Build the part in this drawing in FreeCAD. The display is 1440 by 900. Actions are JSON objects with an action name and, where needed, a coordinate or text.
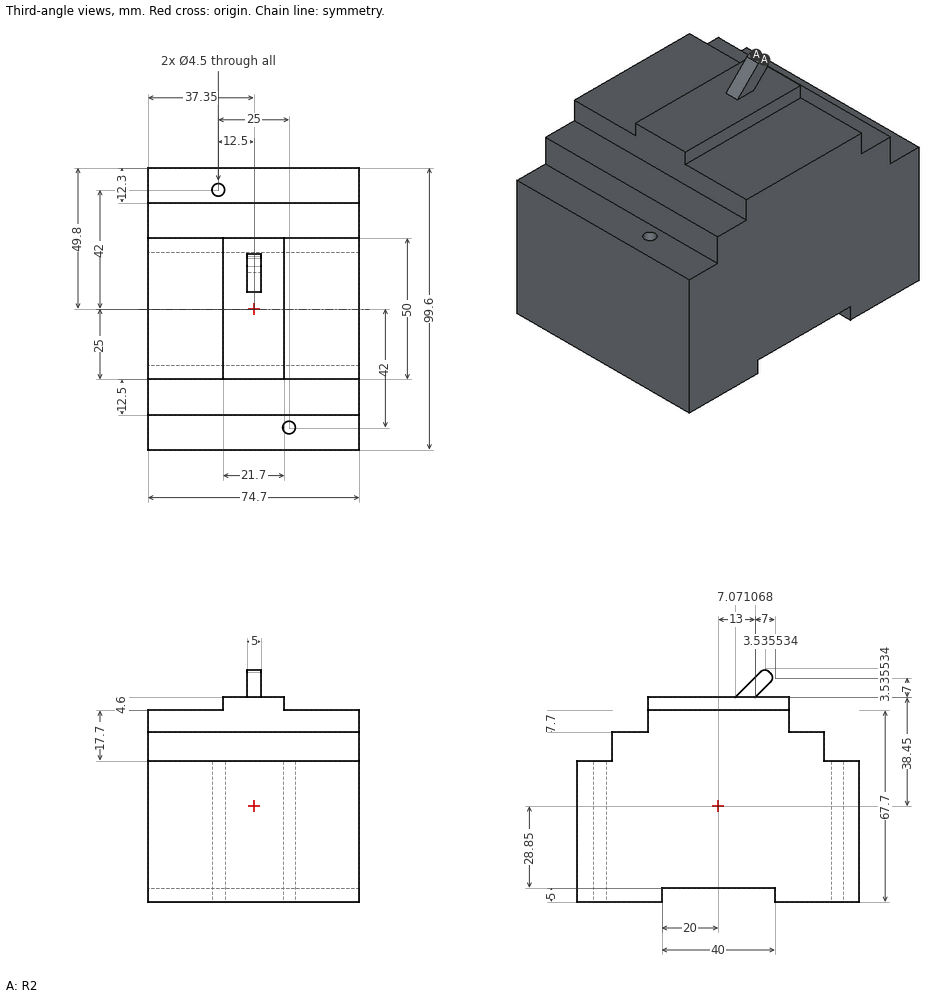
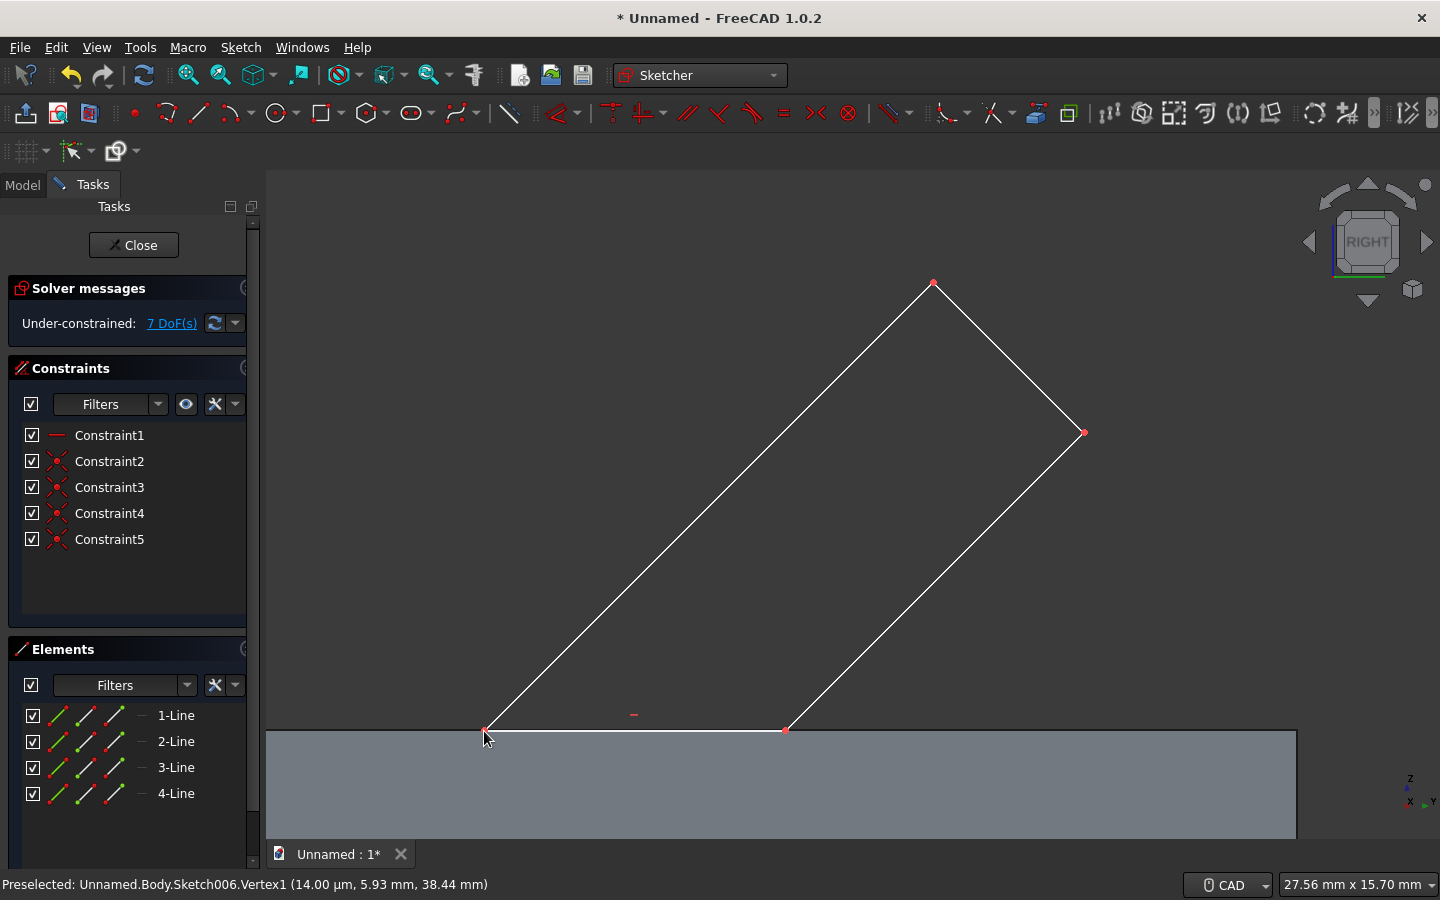
{"action": "left_click", "coordinate": [556, 114]}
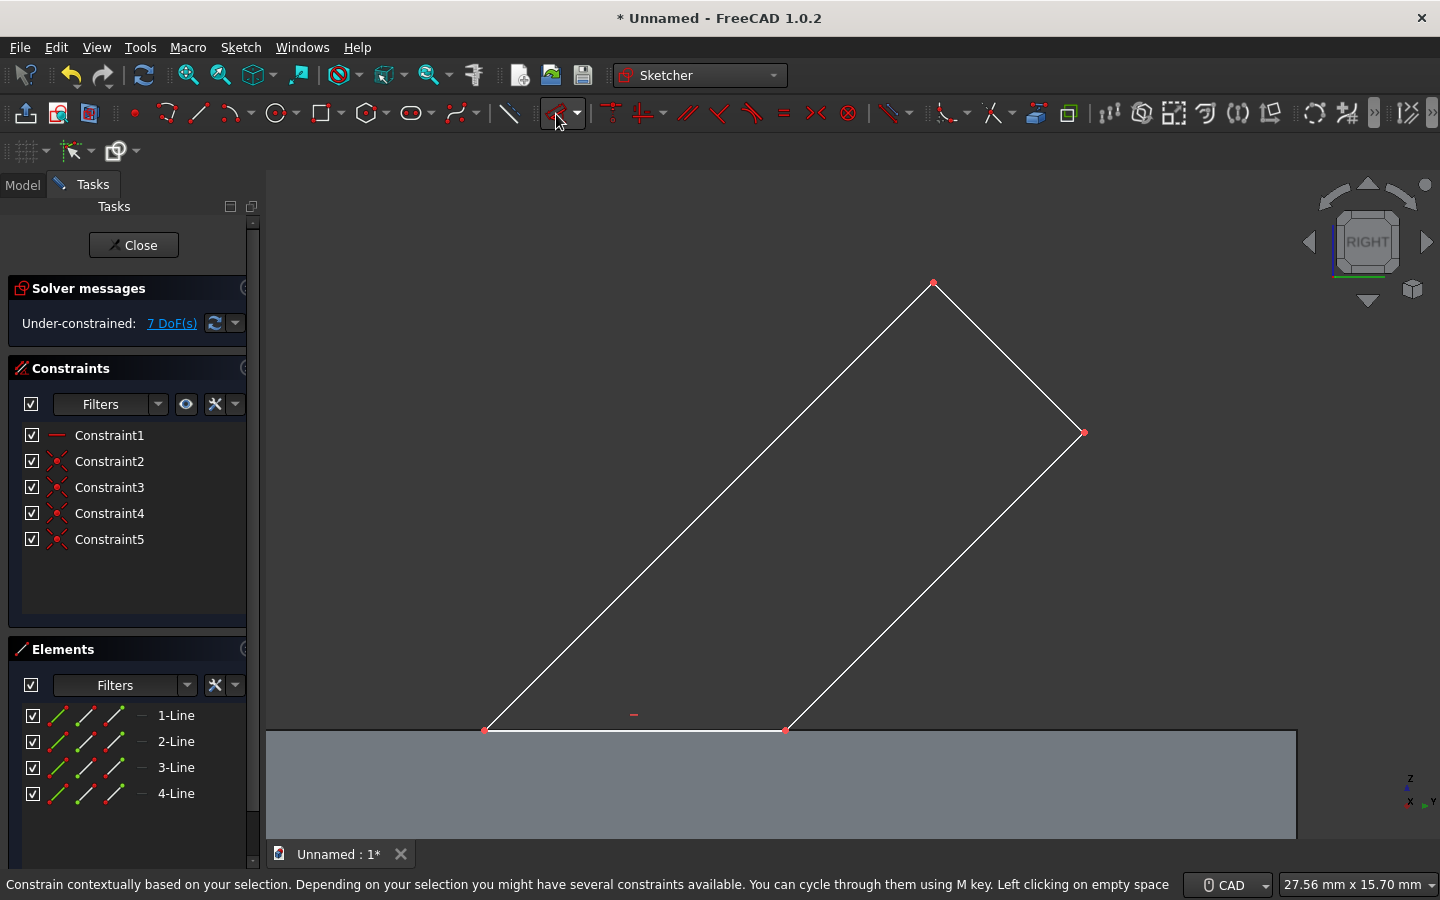
{"action": "left_click", "coordinate": [875, 642]}
{"action": "left_click", "coordinate": [934, 765]}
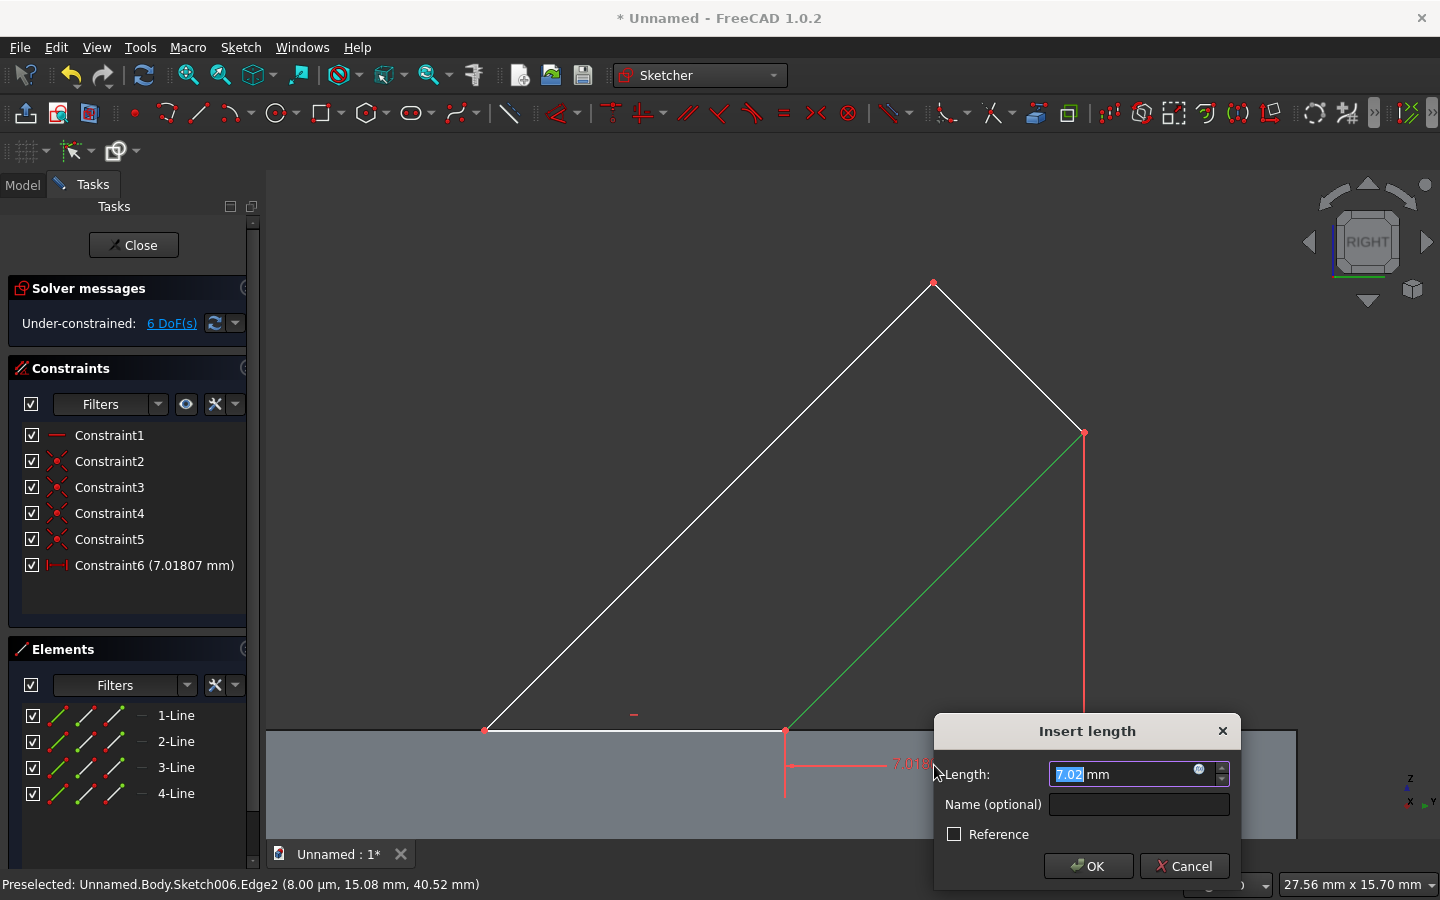
{"action": "type", "text": "7"}
{"action": "key", "text": "Return"}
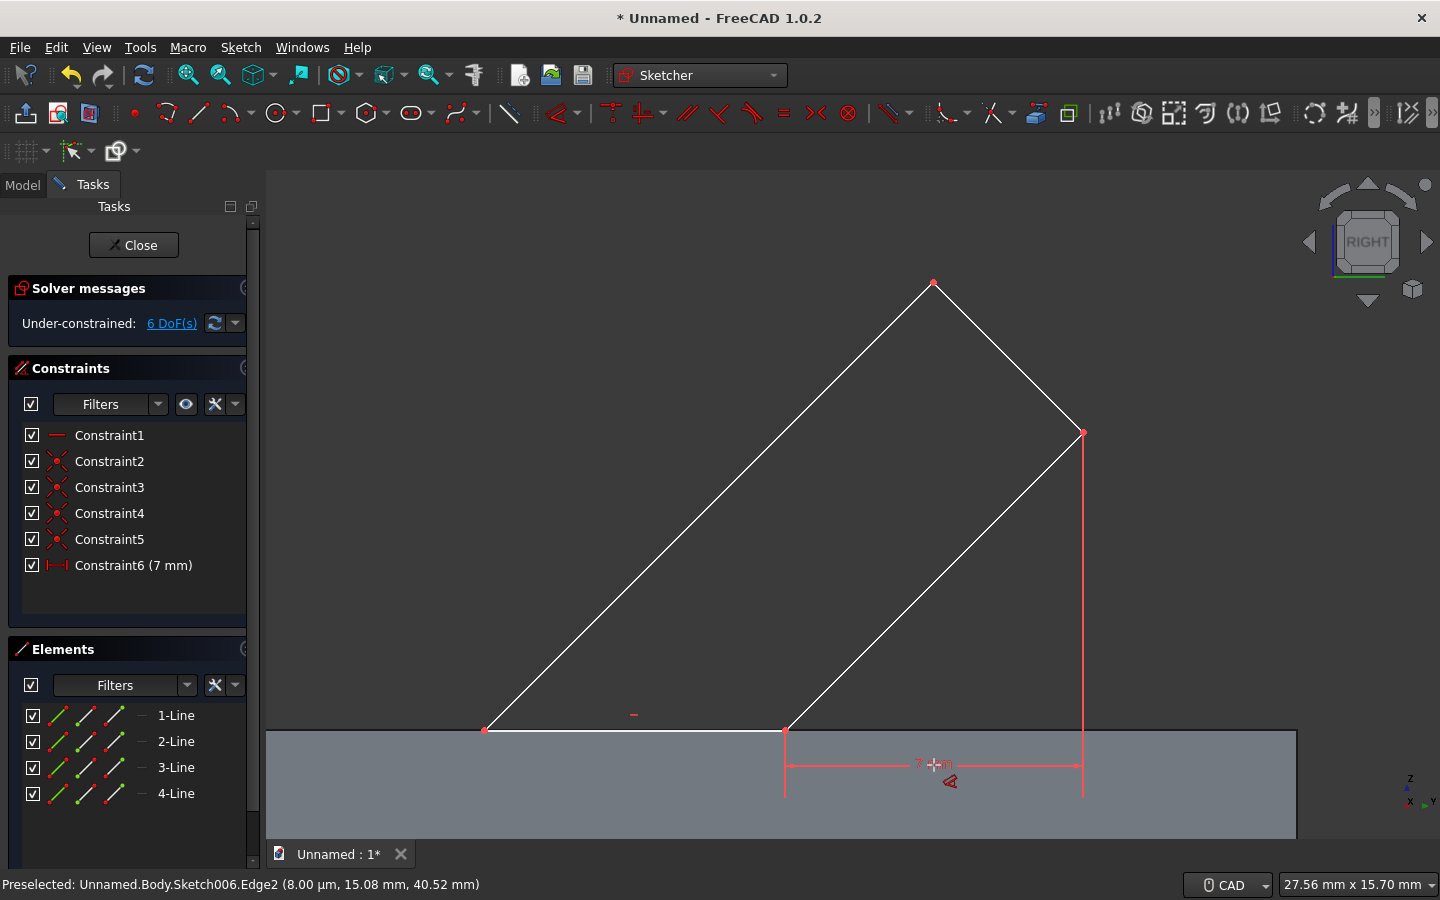
{"action": "left_click", "coordinate": [874, 642]}
{"action": "left_click", "coordinate": [1117, 582]}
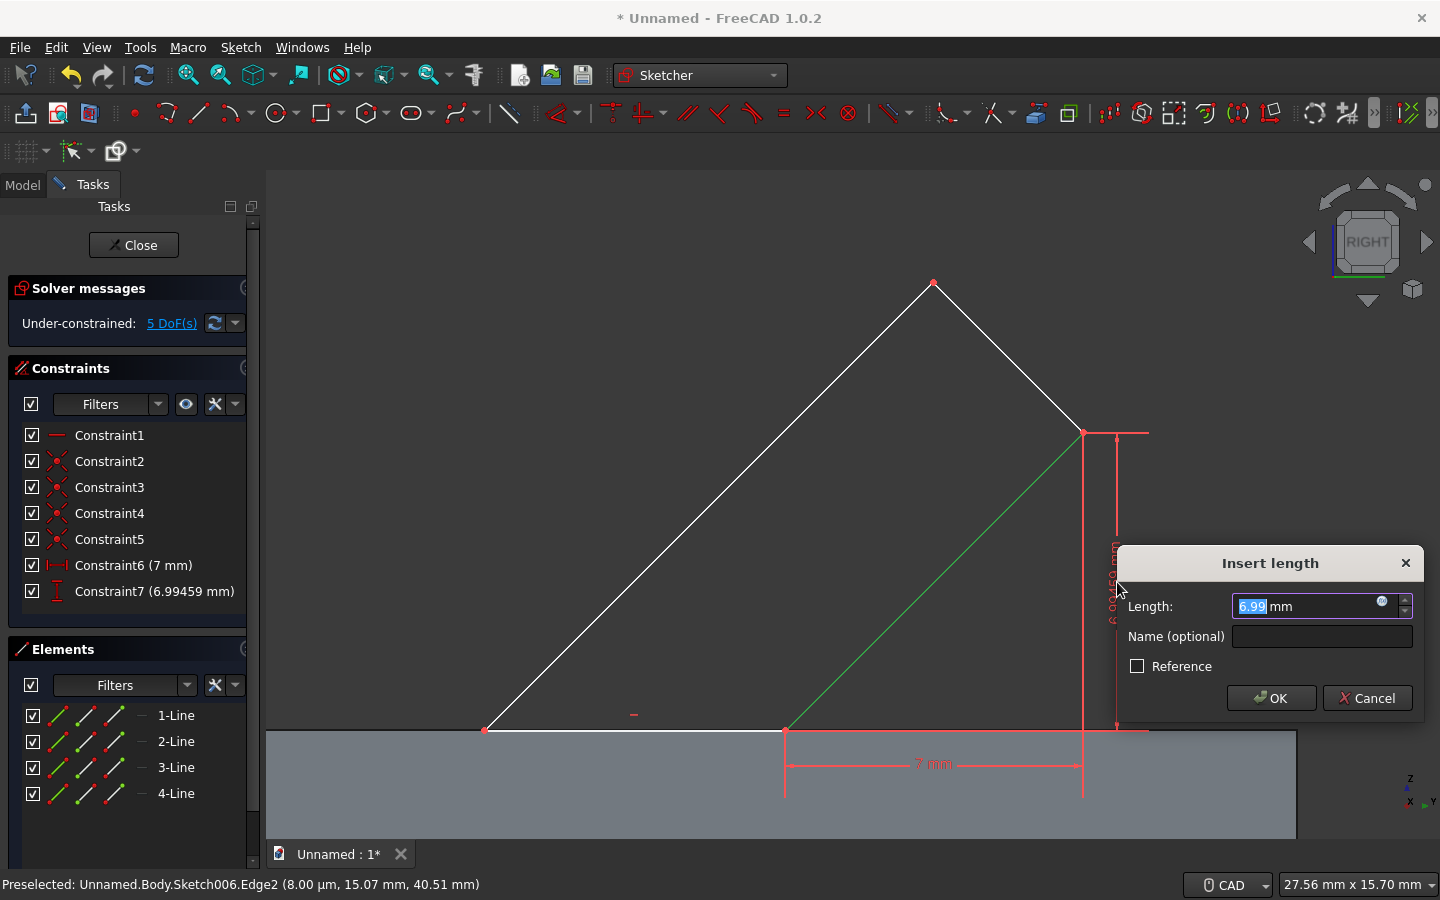
{"action": "type", "text": "7"}
{"action": "key", "text": "Return"}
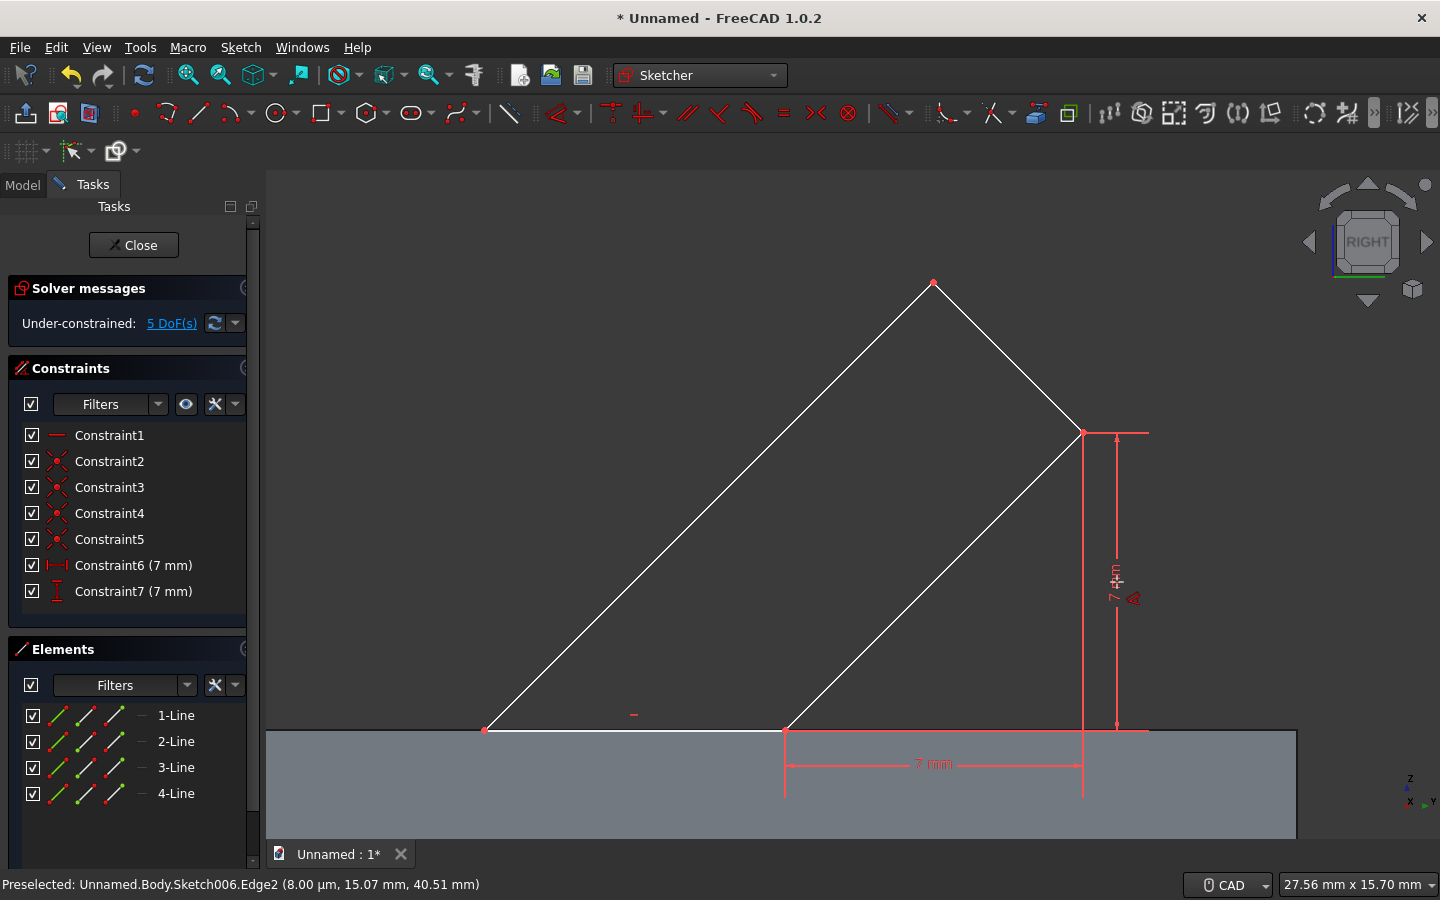
{"action": "left_click", "coordinate": [785, 731]}
{"action": "left_click", "coordinate": [539, 697]}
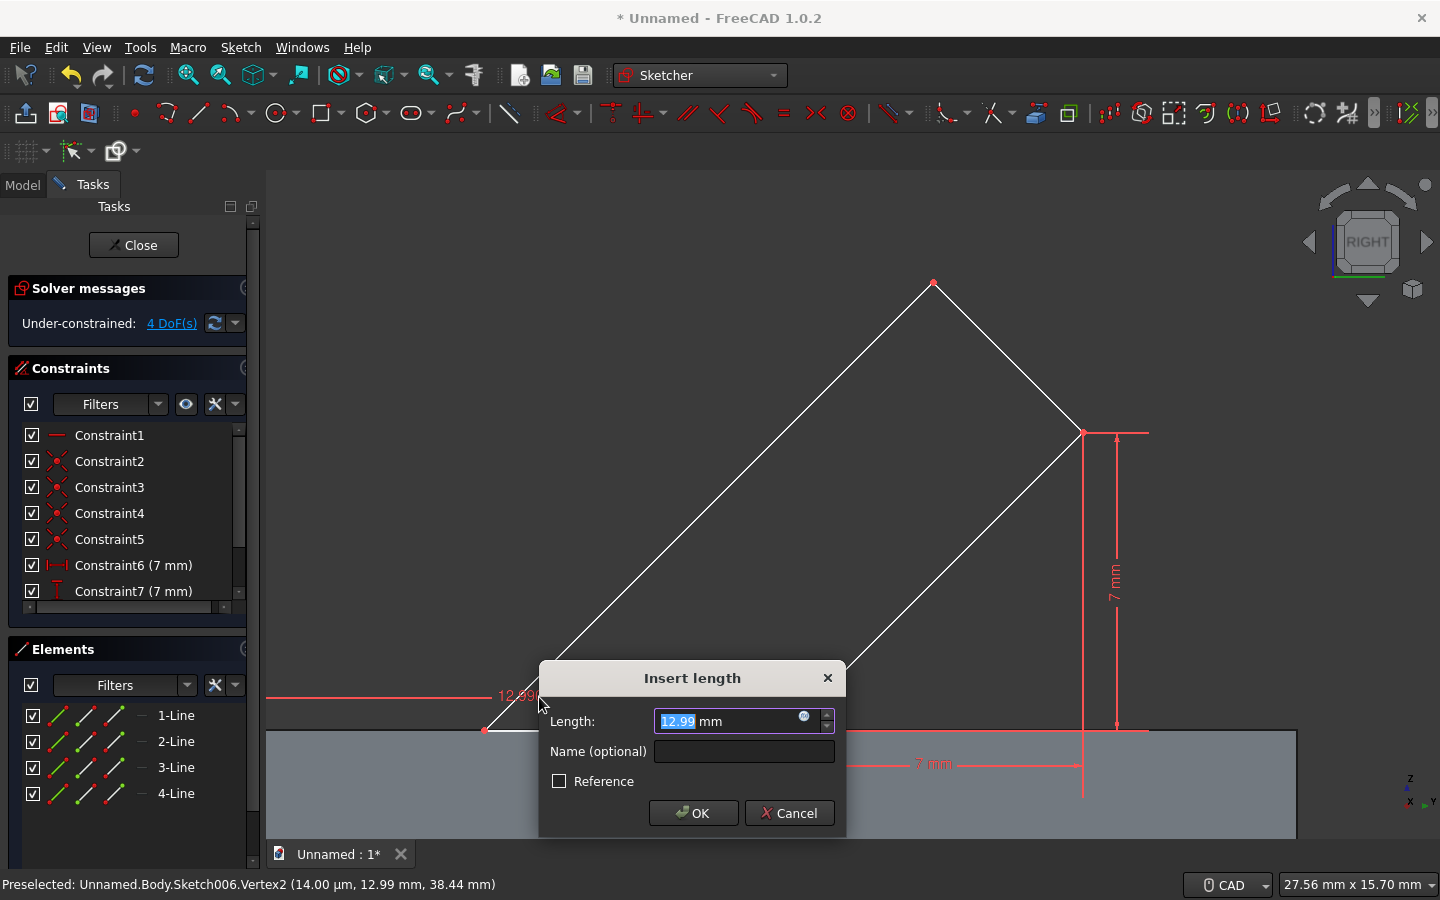
{"action": "type", "text": "13"}
{"action": "key", "text": "Return"}